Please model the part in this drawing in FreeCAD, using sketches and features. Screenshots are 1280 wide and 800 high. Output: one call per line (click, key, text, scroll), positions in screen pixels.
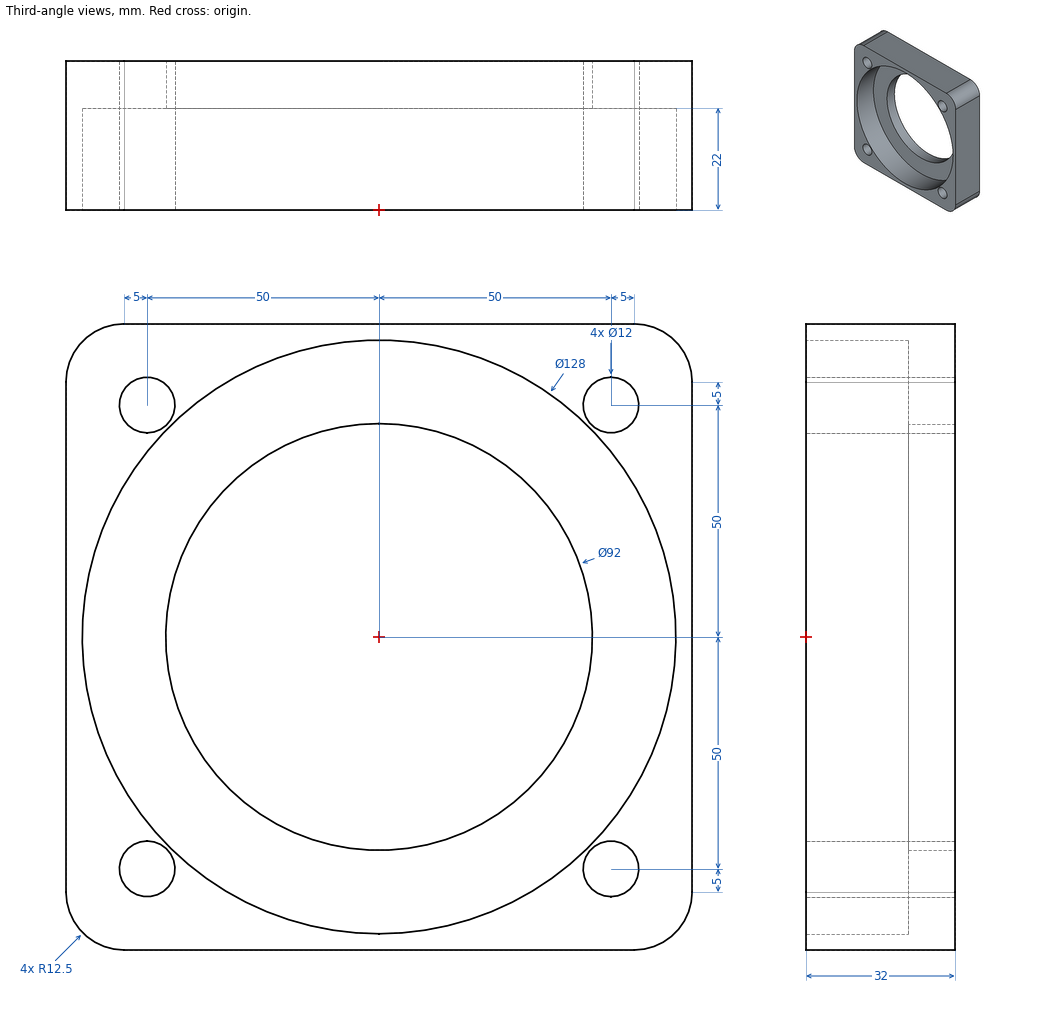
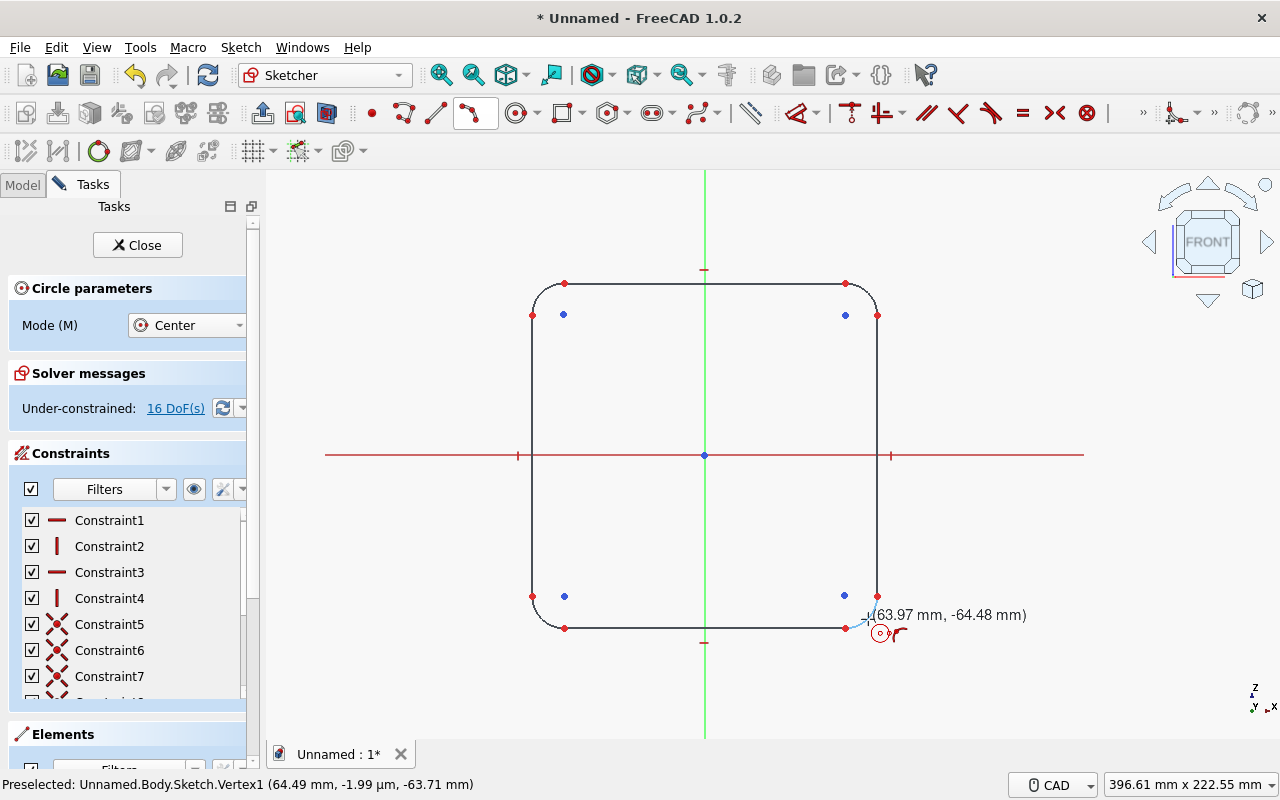
scroll(833, 327, up, 2)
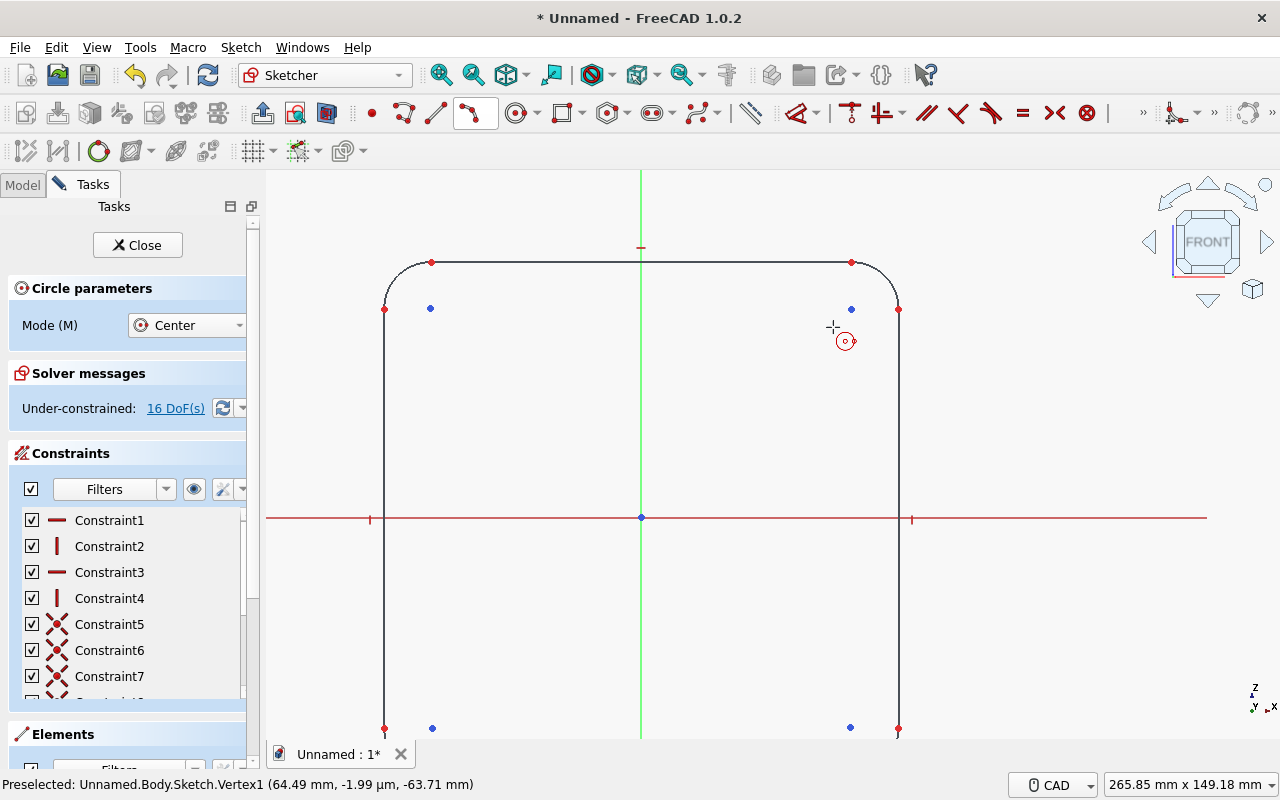
click(832, 327)
click(816, 311)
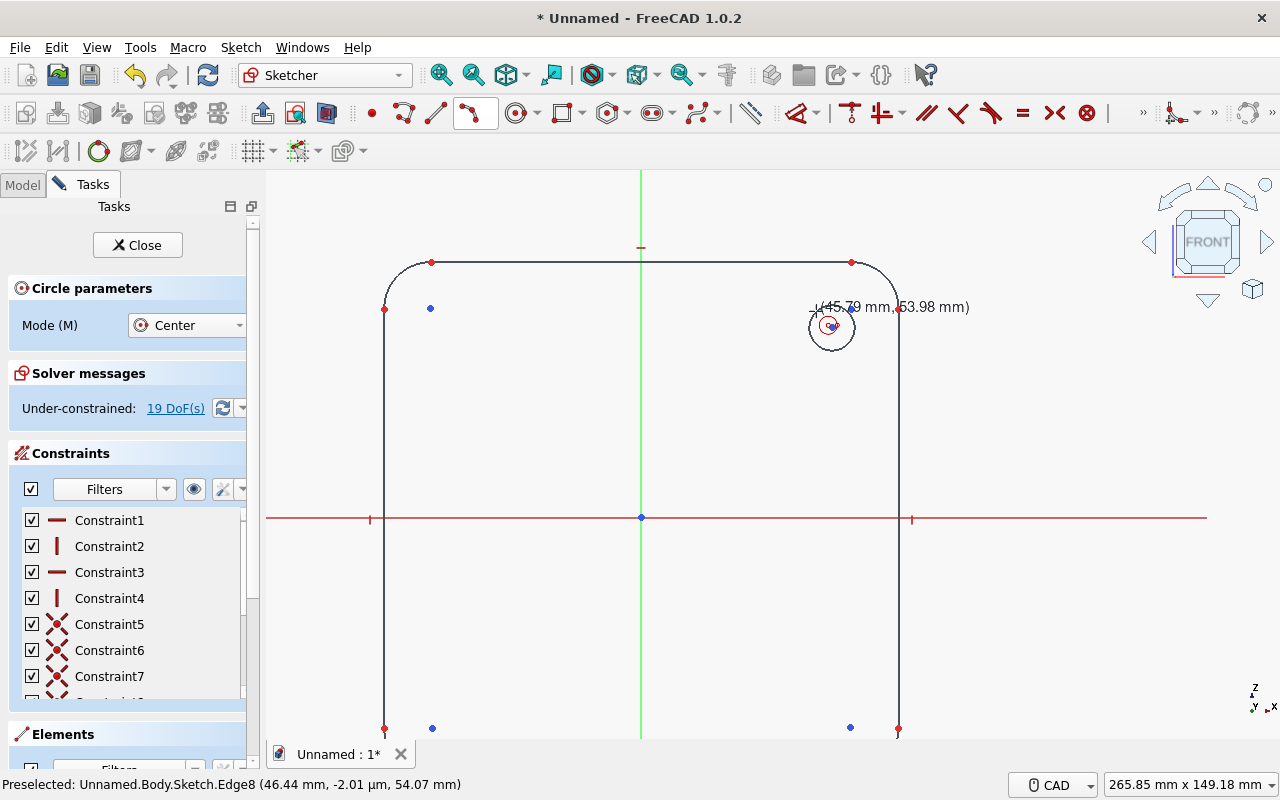
click(451, 327)
click(467, 311)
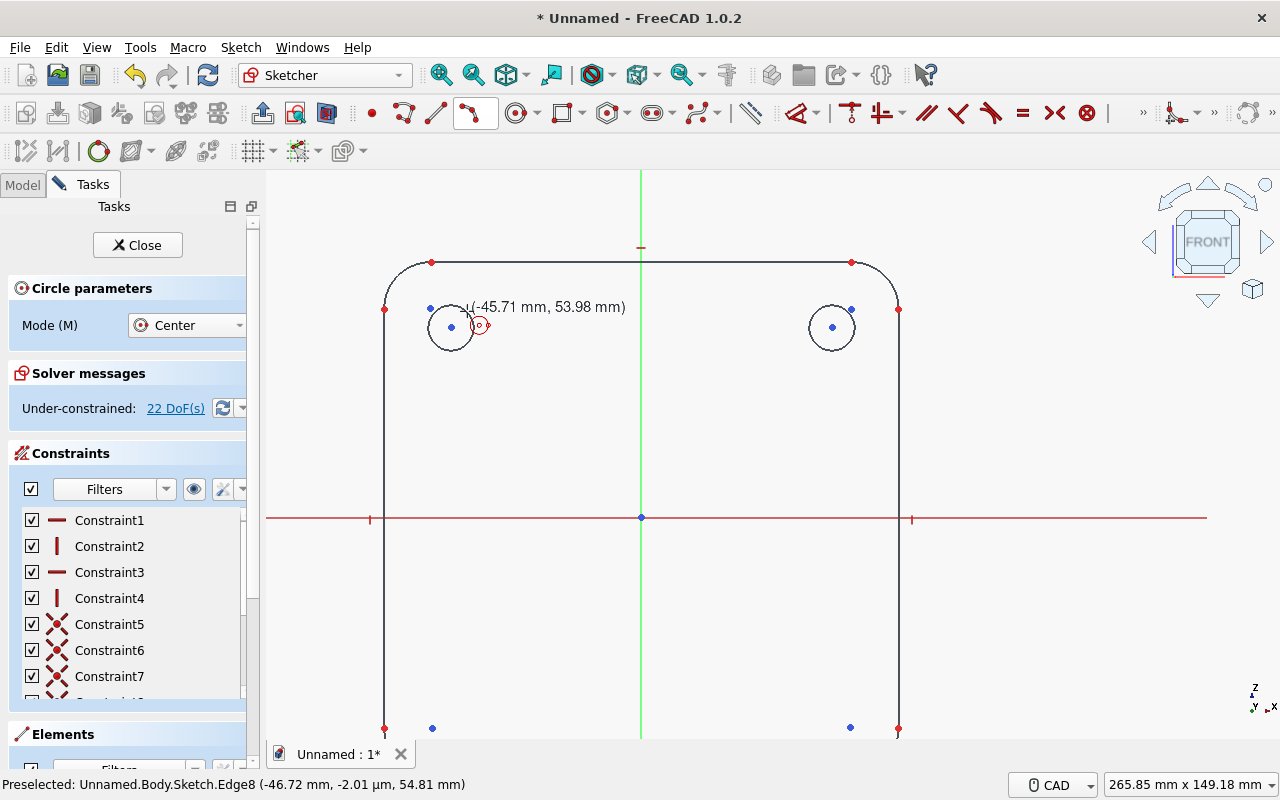
click(832, 709)
click(848, 692)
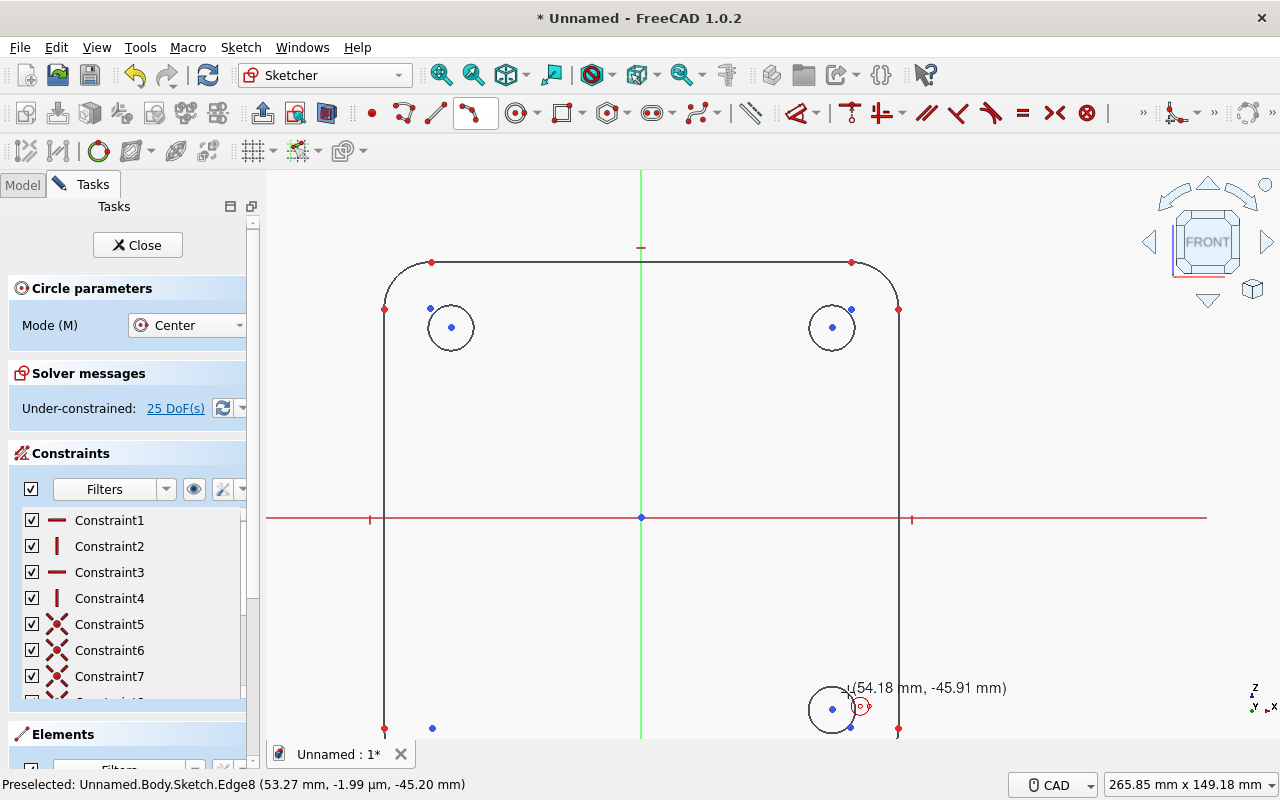
click(451, 709)
click(467, 692)
key(Escape)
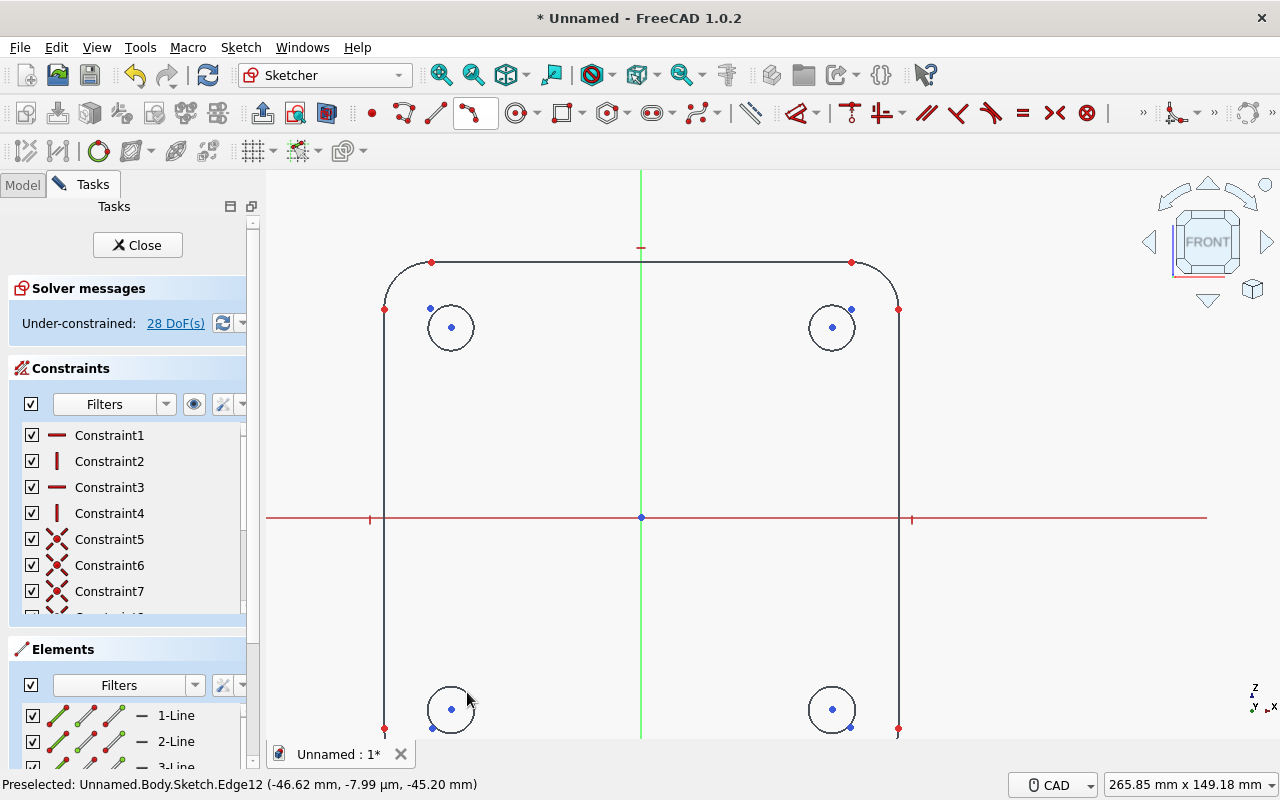
scroll(833, 326, down, 2)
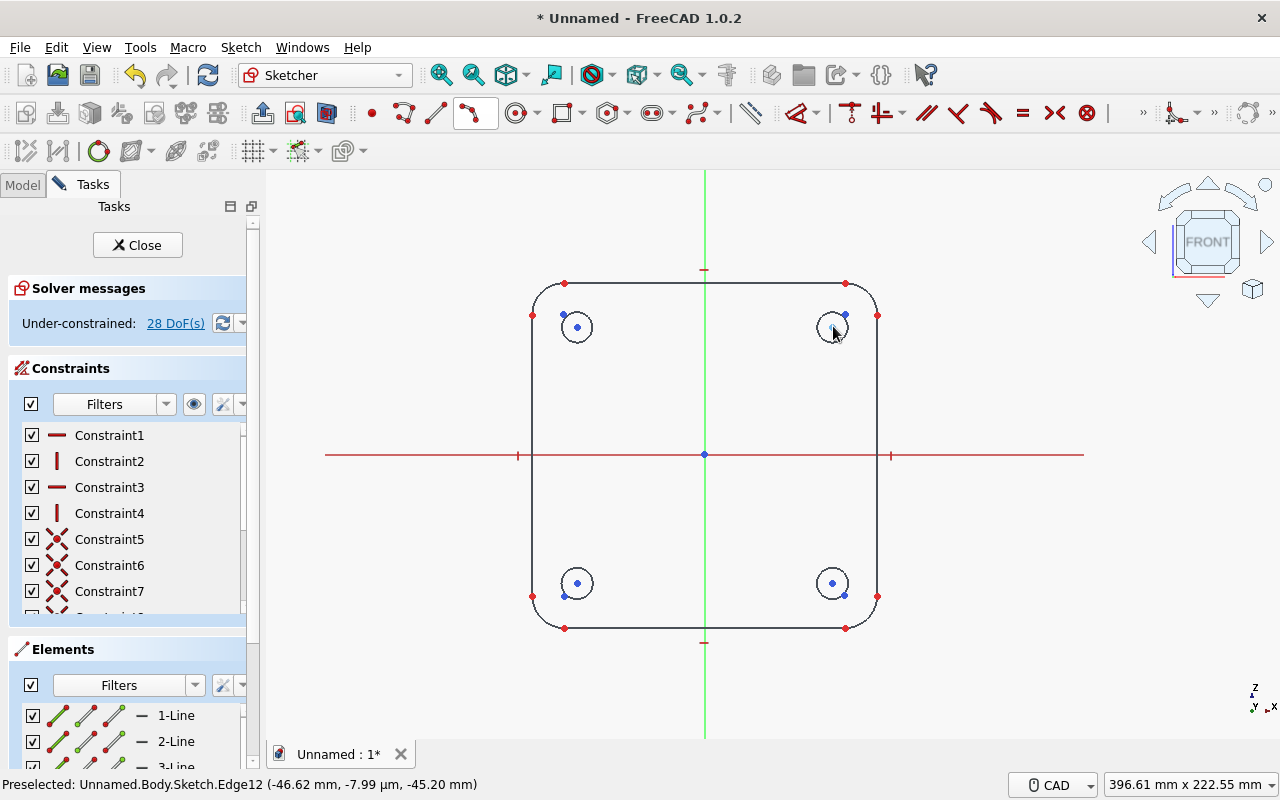
click(761, 628)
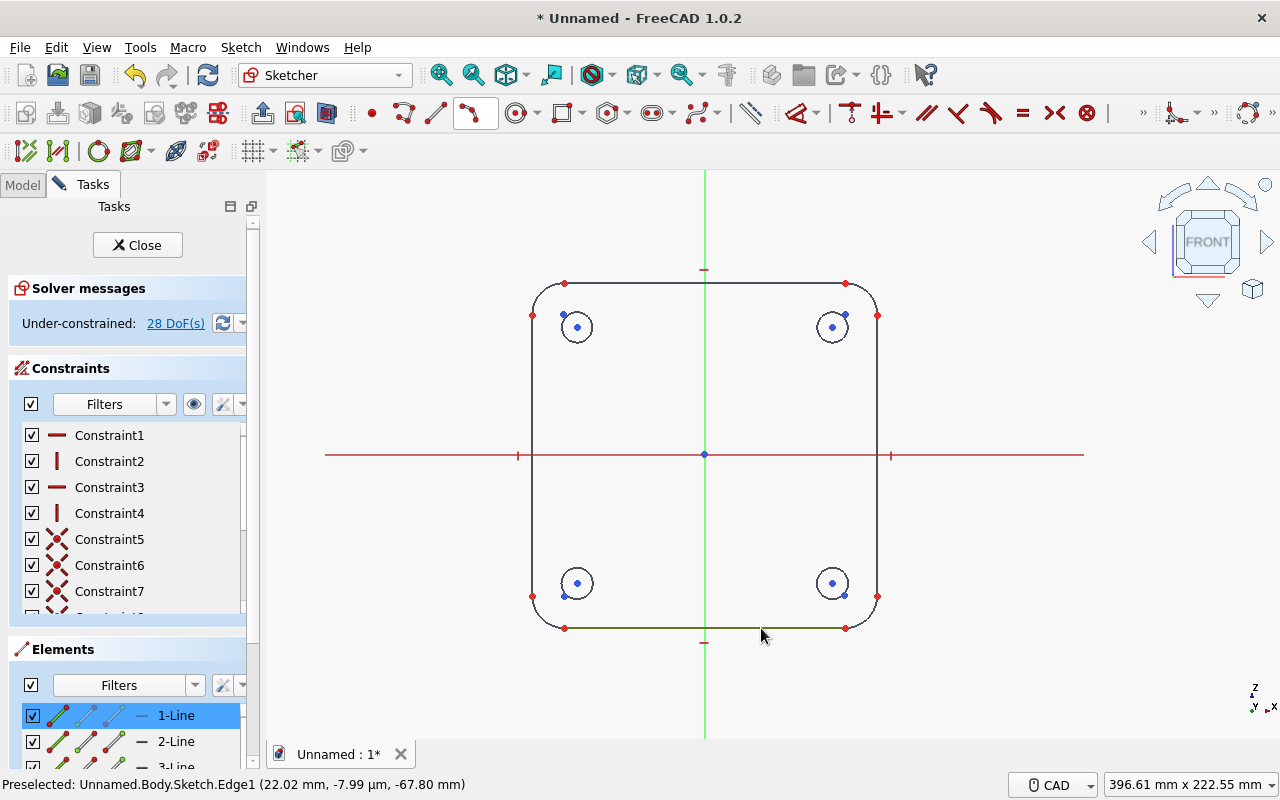
click(536, 611)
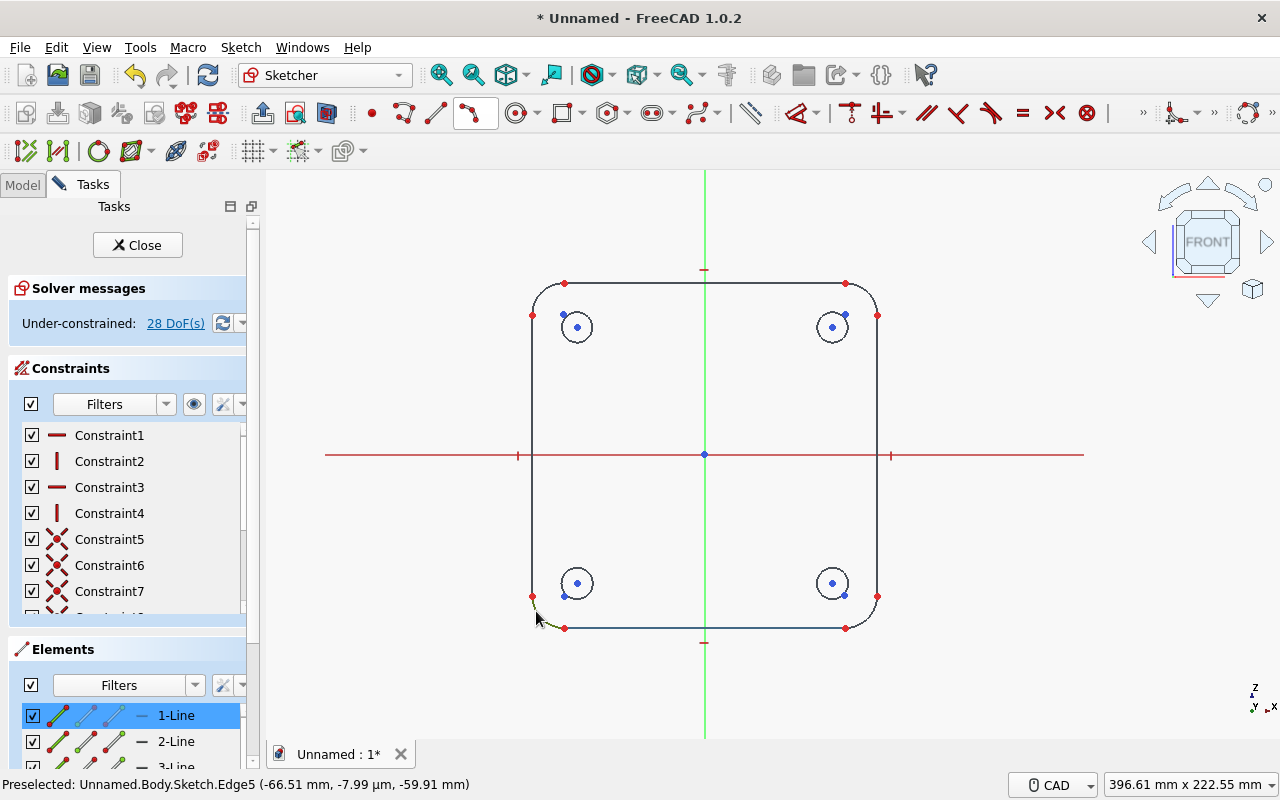
key(t)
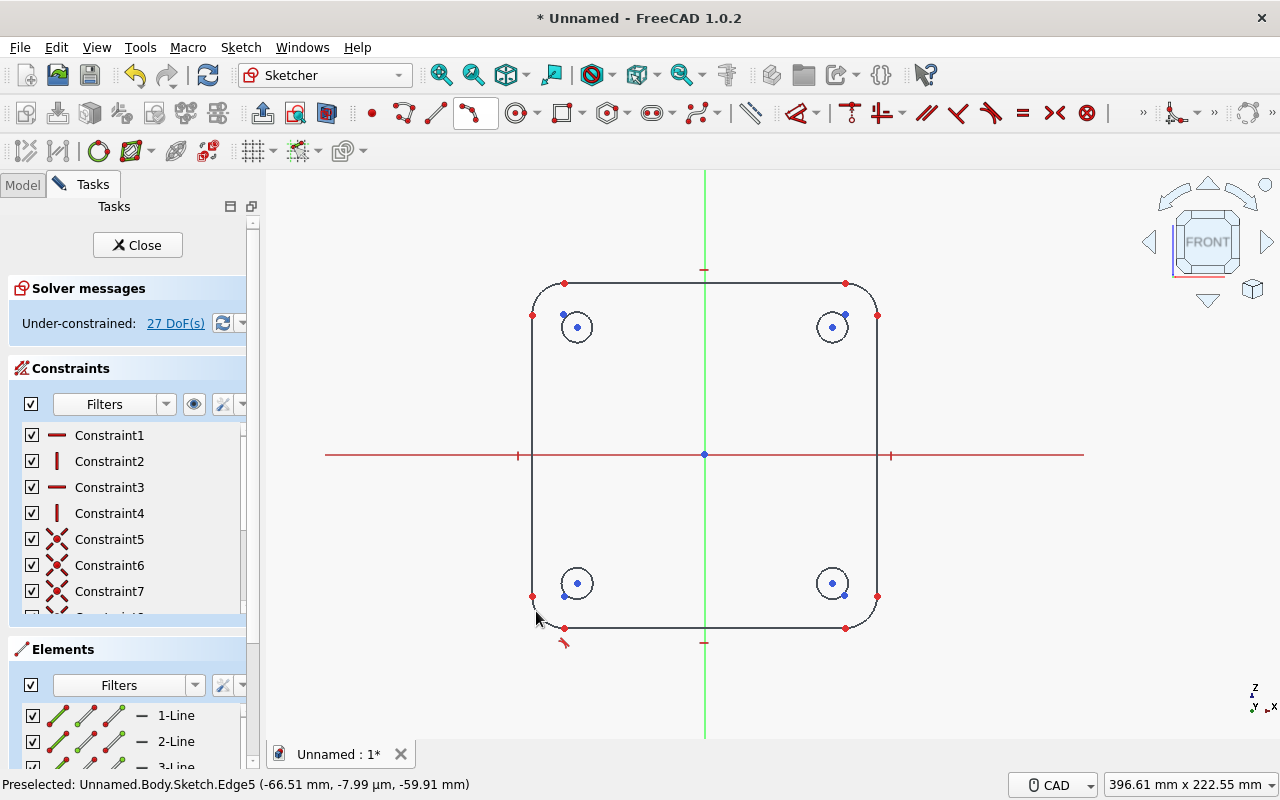
click(761, 628)